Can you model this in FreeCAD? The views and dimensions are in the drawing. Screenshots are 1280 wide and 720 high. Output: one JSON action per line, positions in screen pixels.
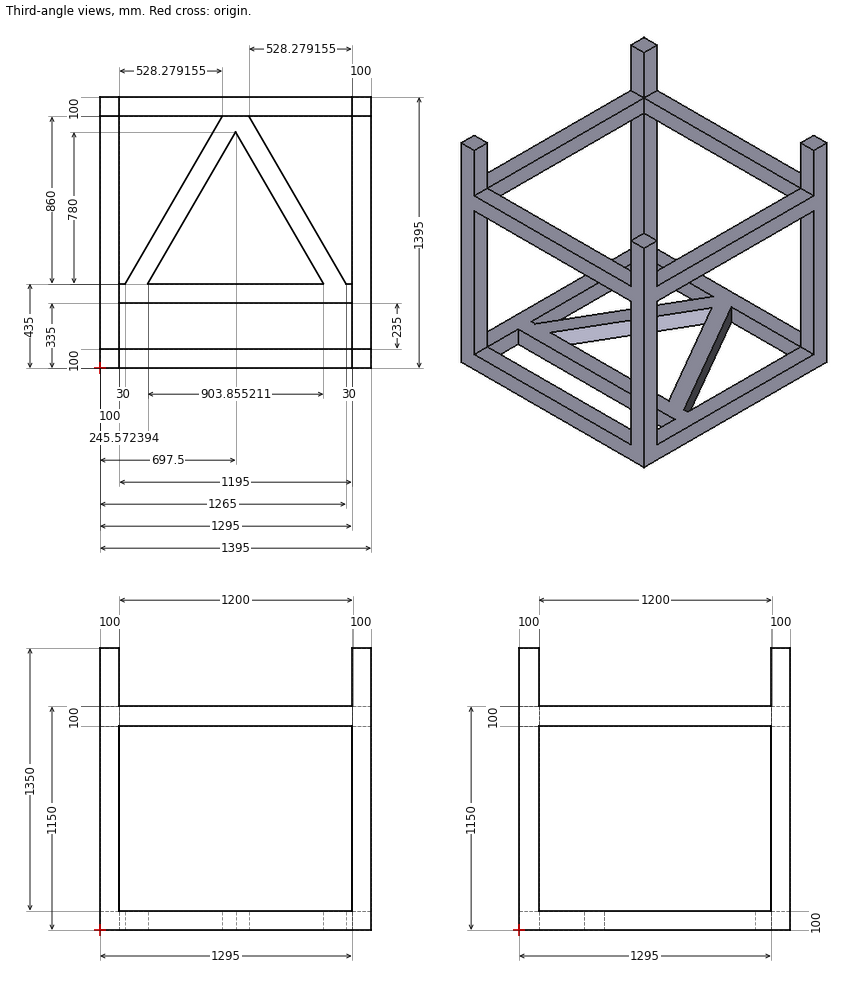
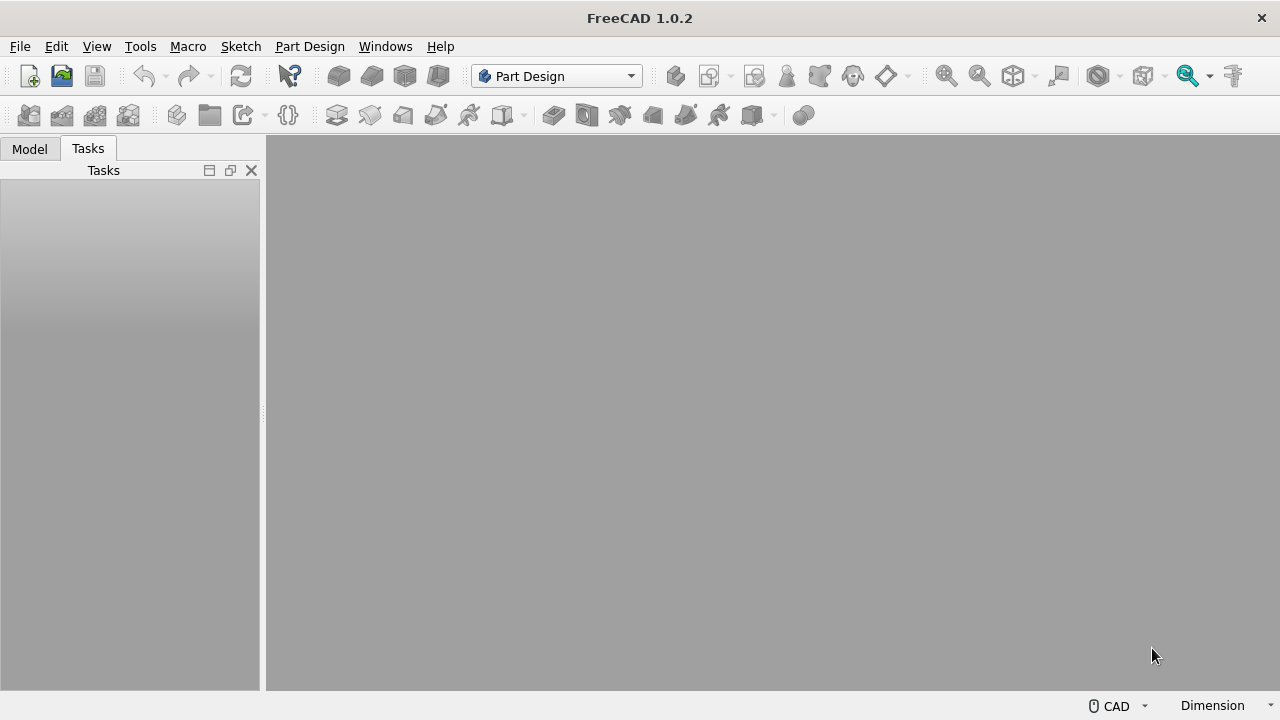
{"action": "left_click", "coordinate": [29, 76]}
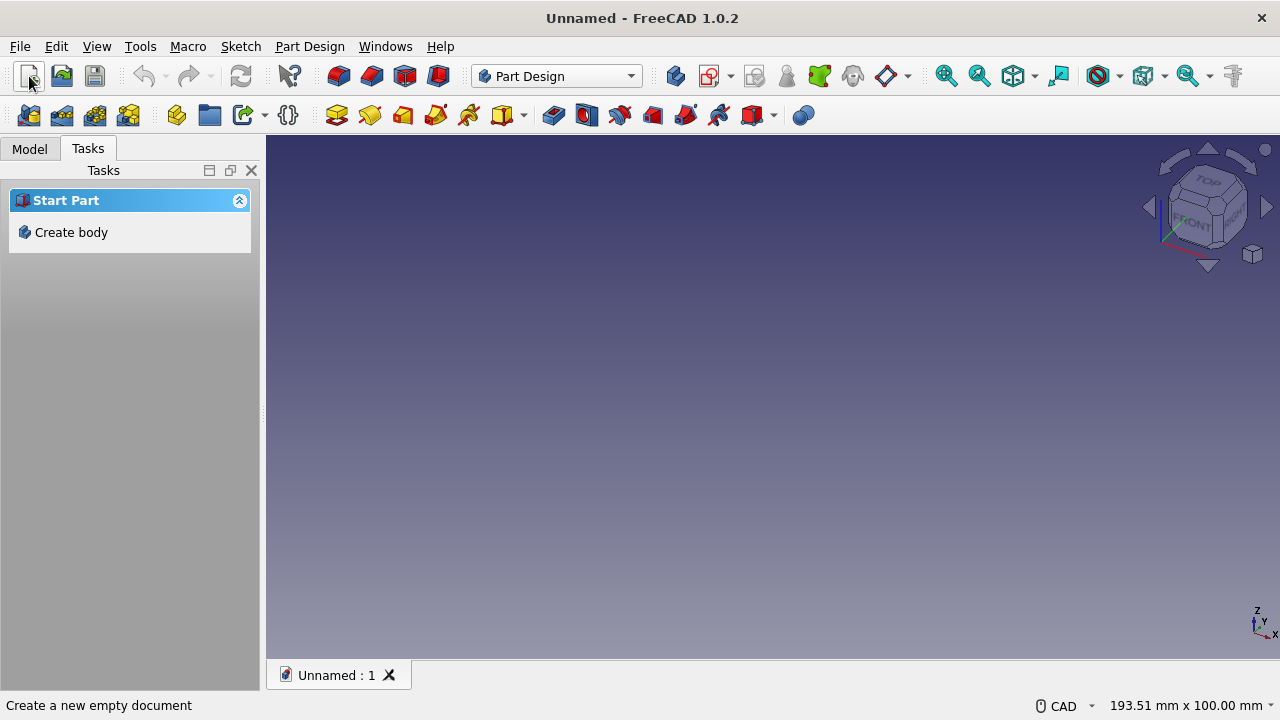
{"action": "left_click", "coordinate": [708, 76]}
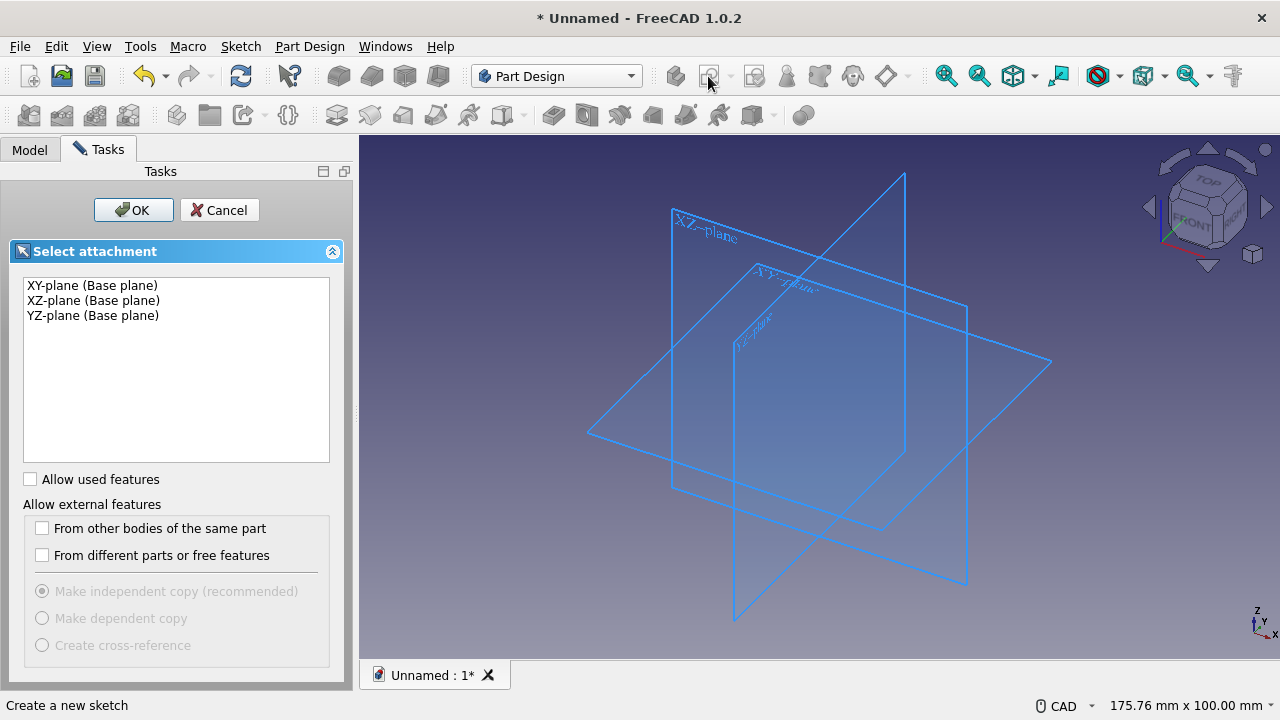
{"action": "left_click", "coordinate": [84, 286]}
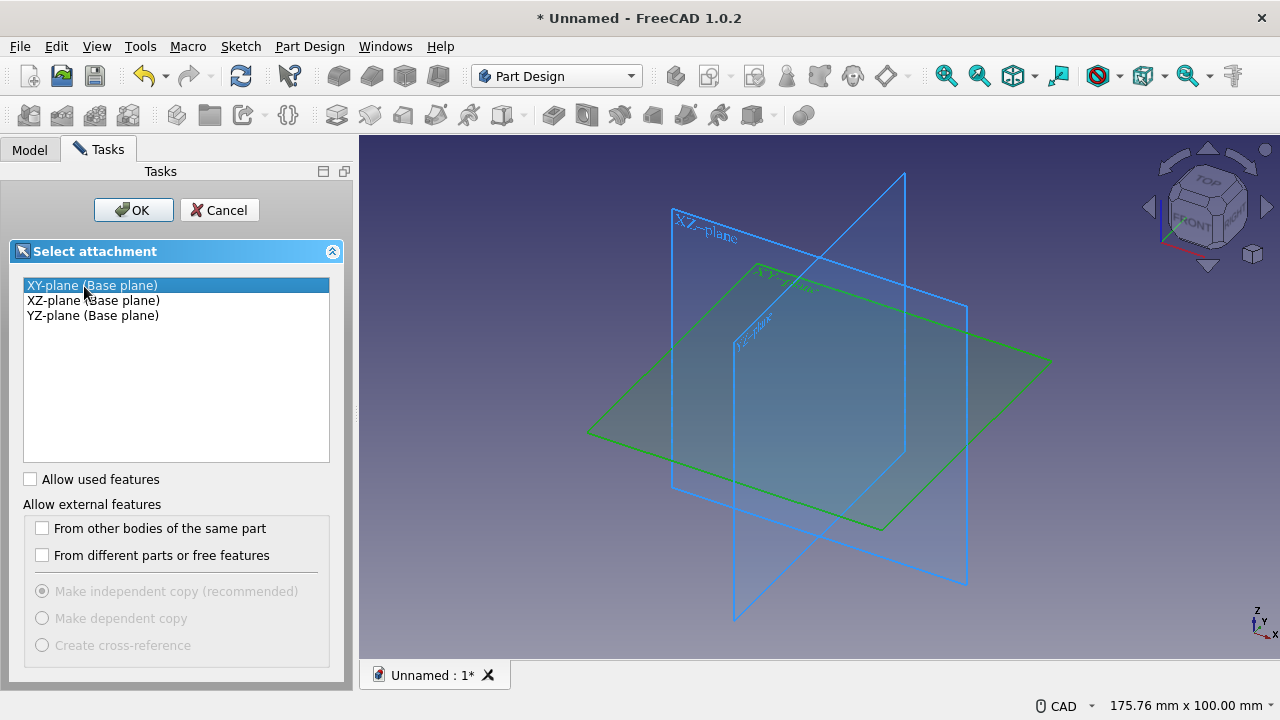
{"action": "left_click", "coordinate": [134, 210]}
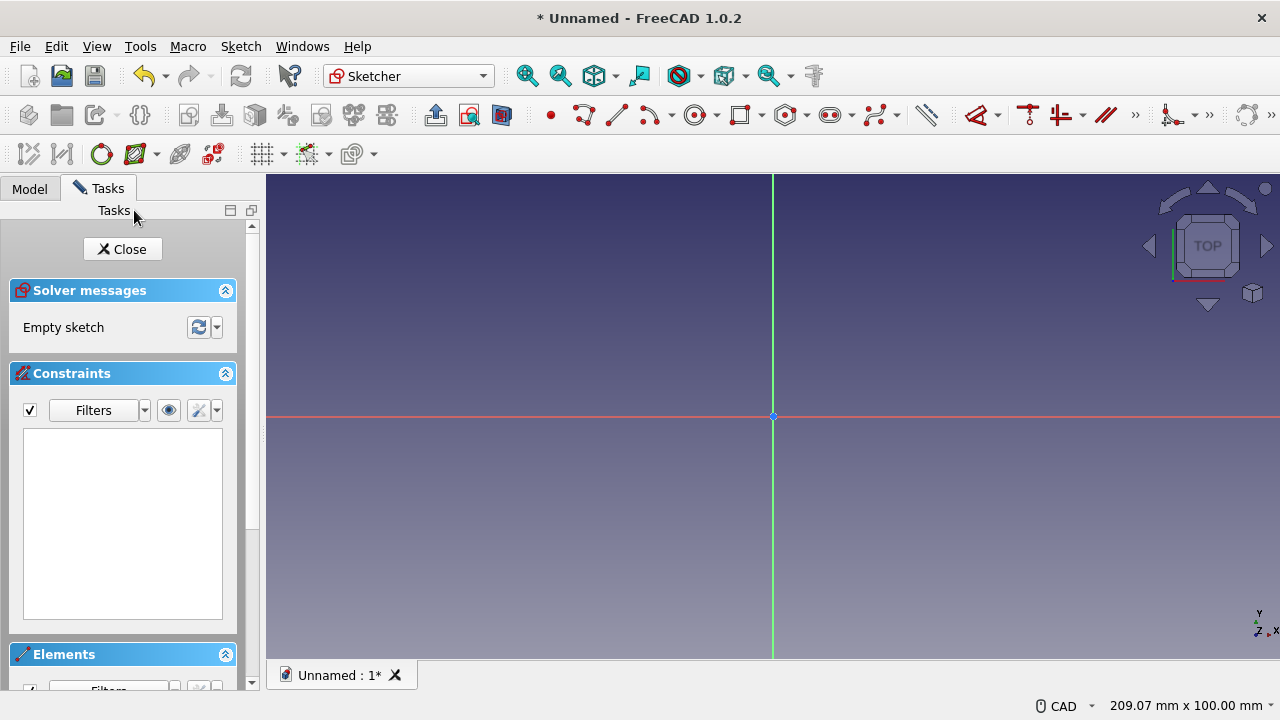
{"action": "scroll", "coordinate": [524, 594], "scroll_direction": "down", "scroll_amount": 15}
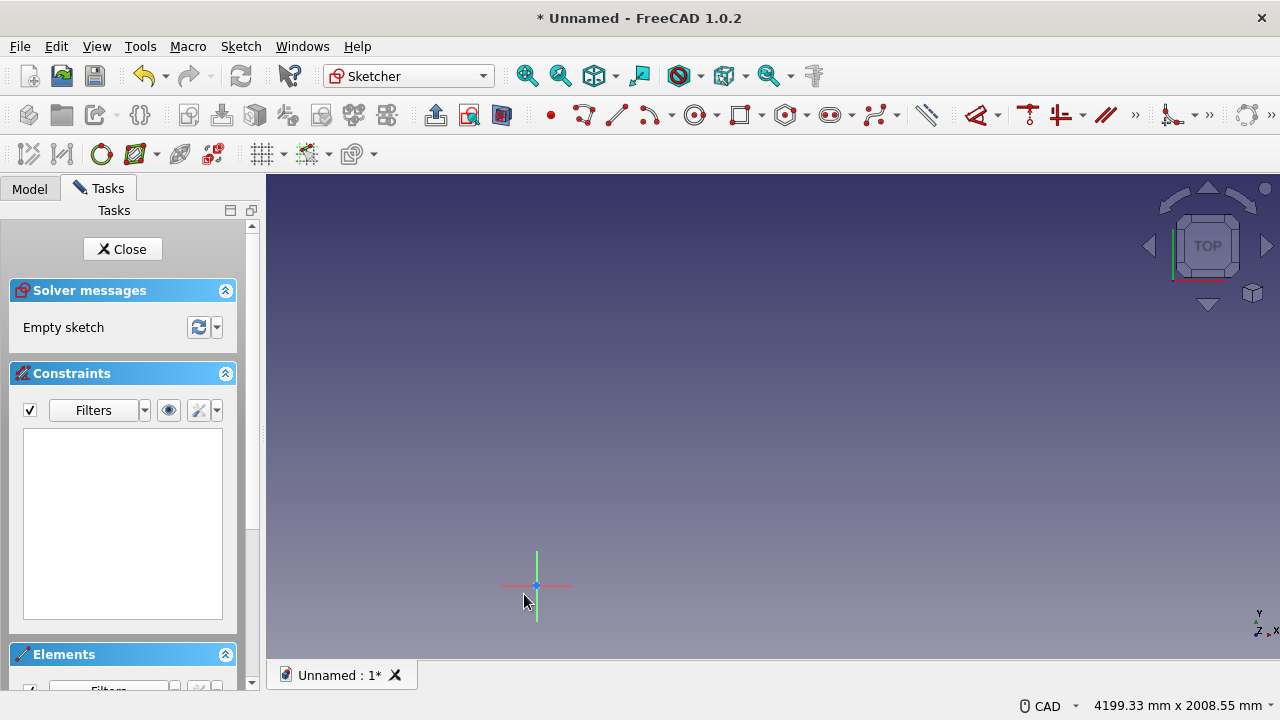
{"action": "left_click", "coordinate": [740, 116]}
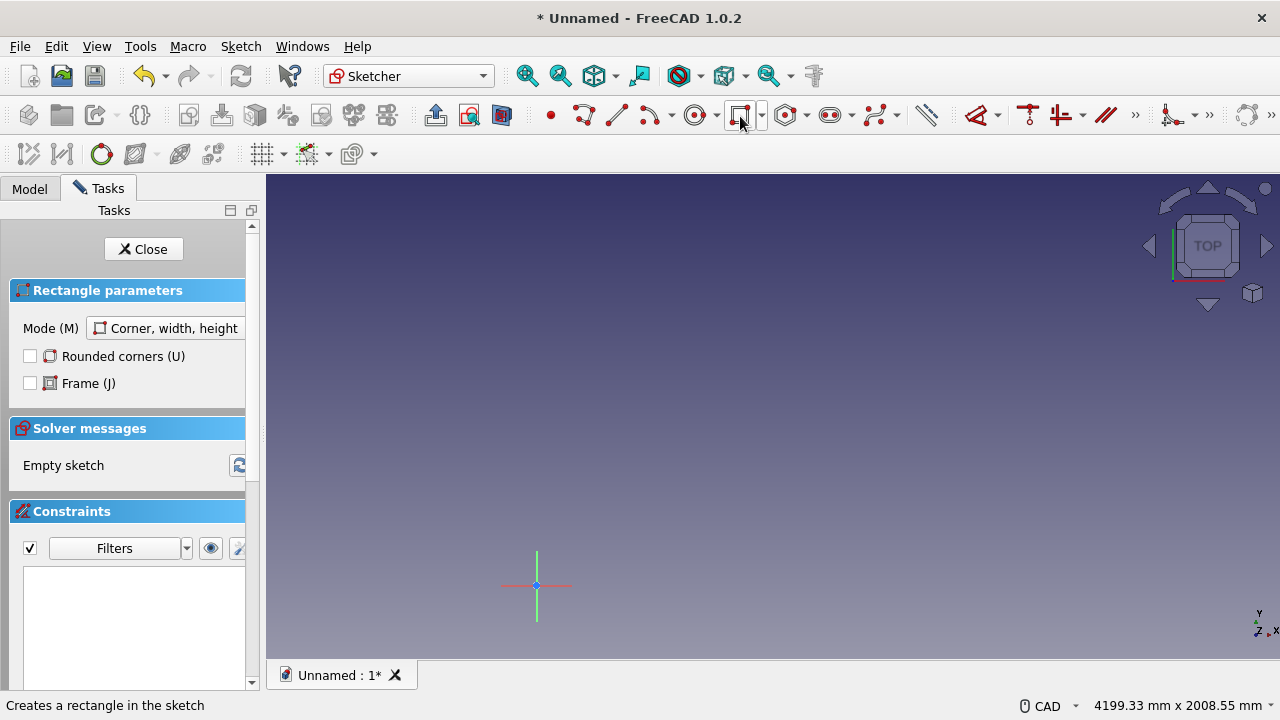
{"action": "left_click", "coordinate": [537, 586]}
{"action": "mouse_move", "coordinate": [873, 249]}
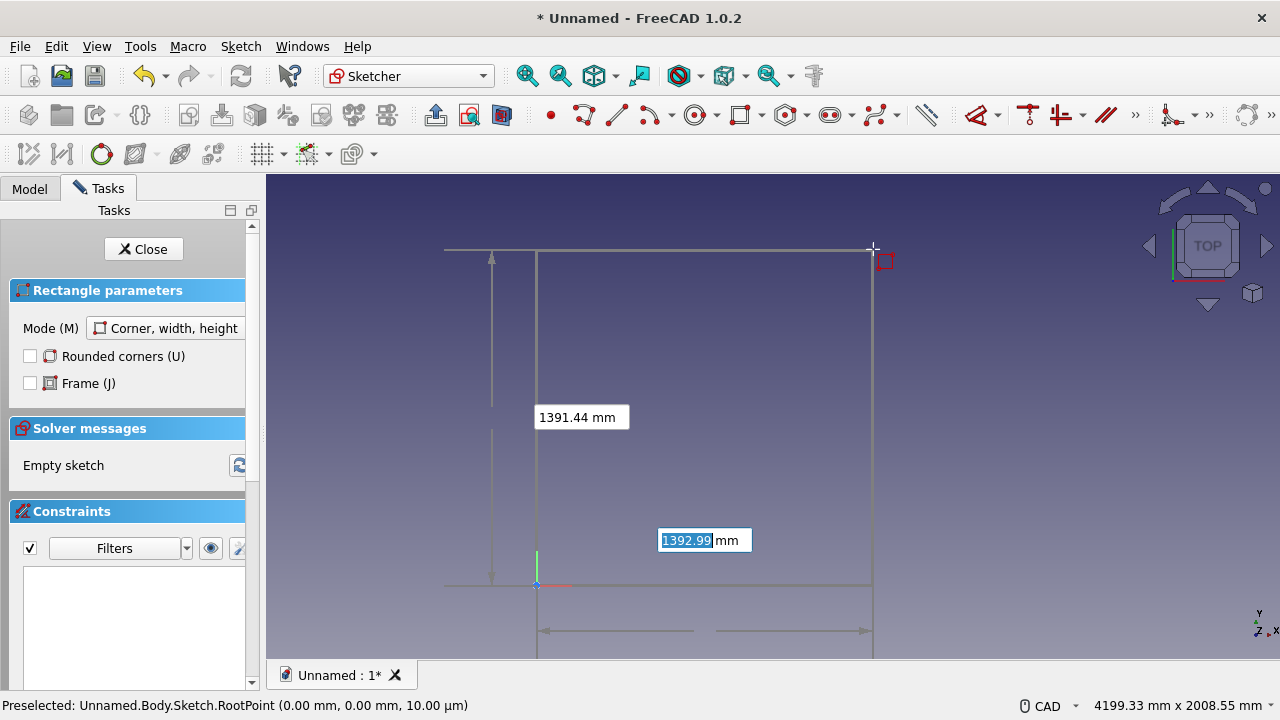
{"action": "type", "text": "1395"}
{"action": "key", "text": "Tab"}
{"action": "type", "text": "1395"}
{"action": "key", "text": "Return"}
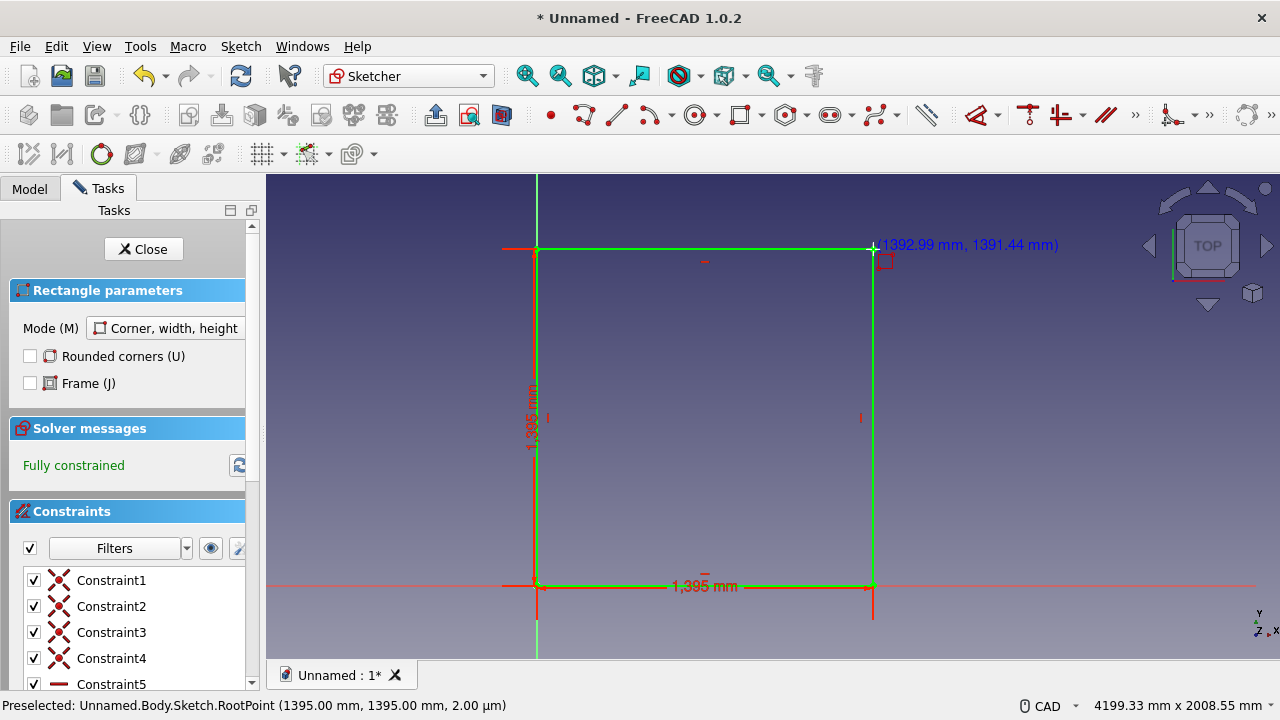
{"action": "left_click", "coordinate": [561, 505]}
{"action": "mouse_move", "coordinate": [849, 562]}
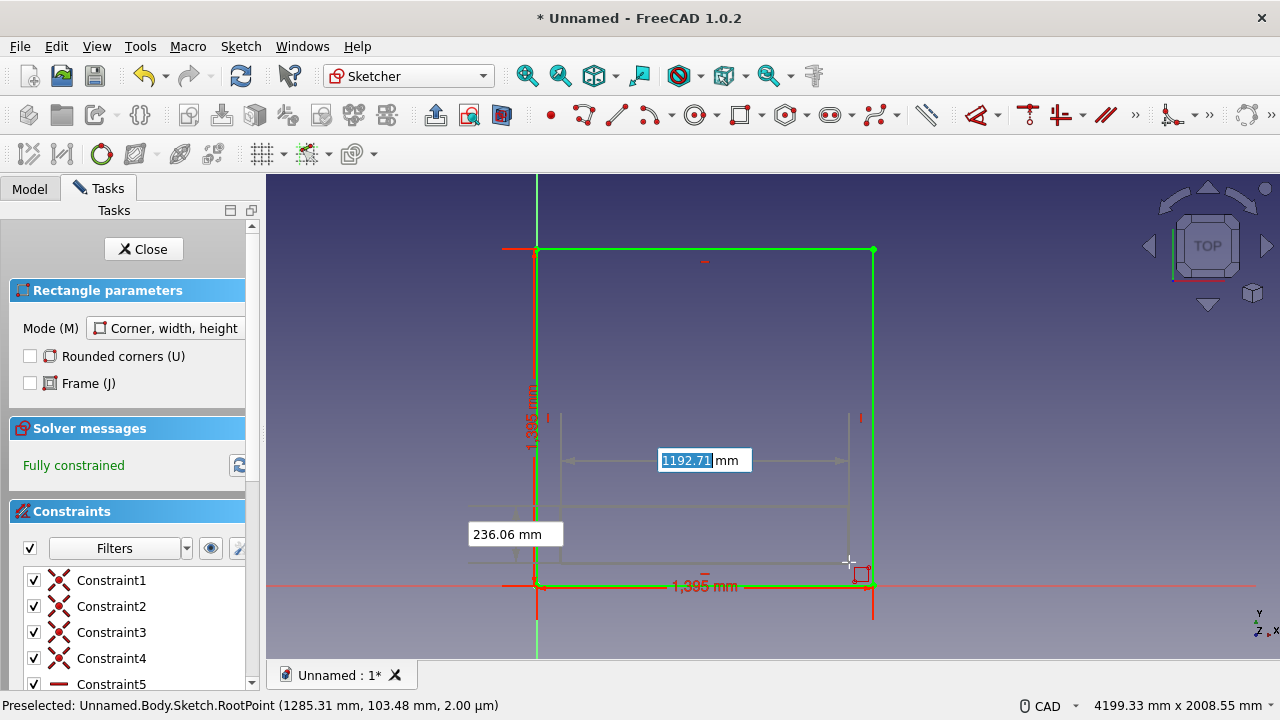
{"action": "type", "text": "1195"}
{"action": "key", "text": "Tab"}
{"action": "type", "text": "235"}
{"action": "key", "text": "Return"}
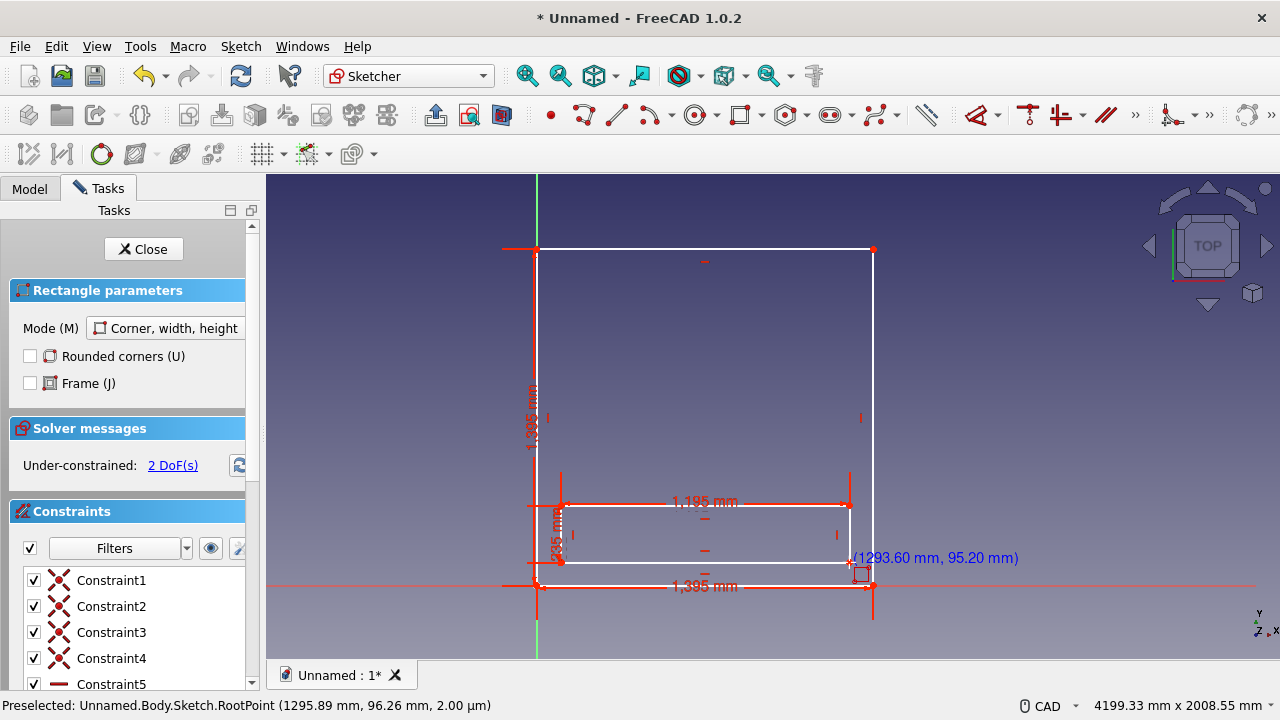
{"action": "left_click", "coordinate": [584, 116]}